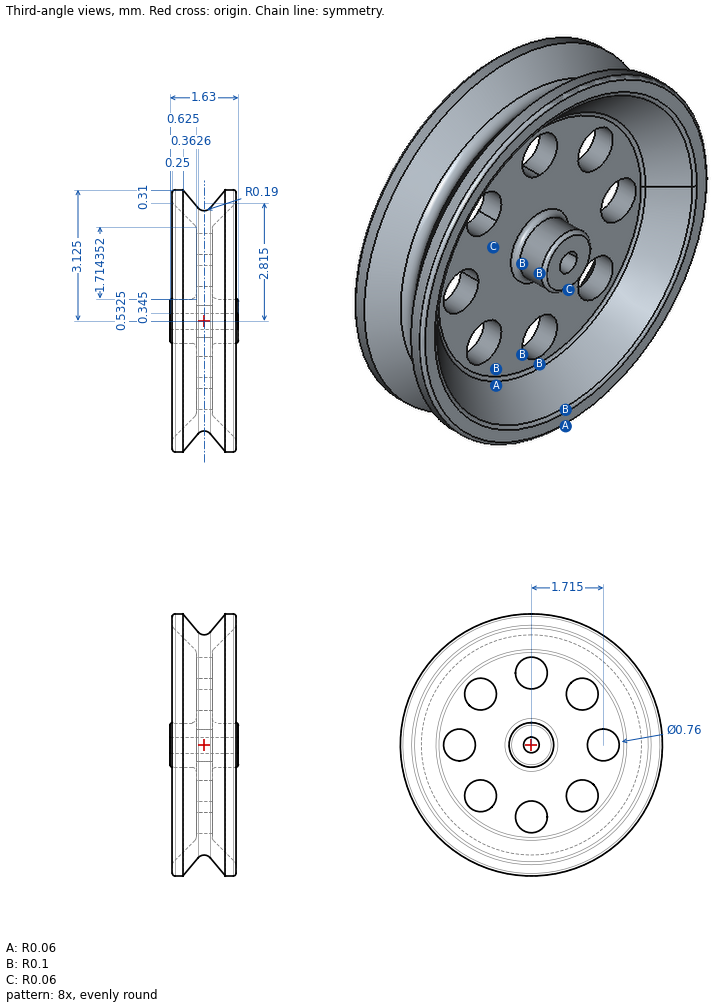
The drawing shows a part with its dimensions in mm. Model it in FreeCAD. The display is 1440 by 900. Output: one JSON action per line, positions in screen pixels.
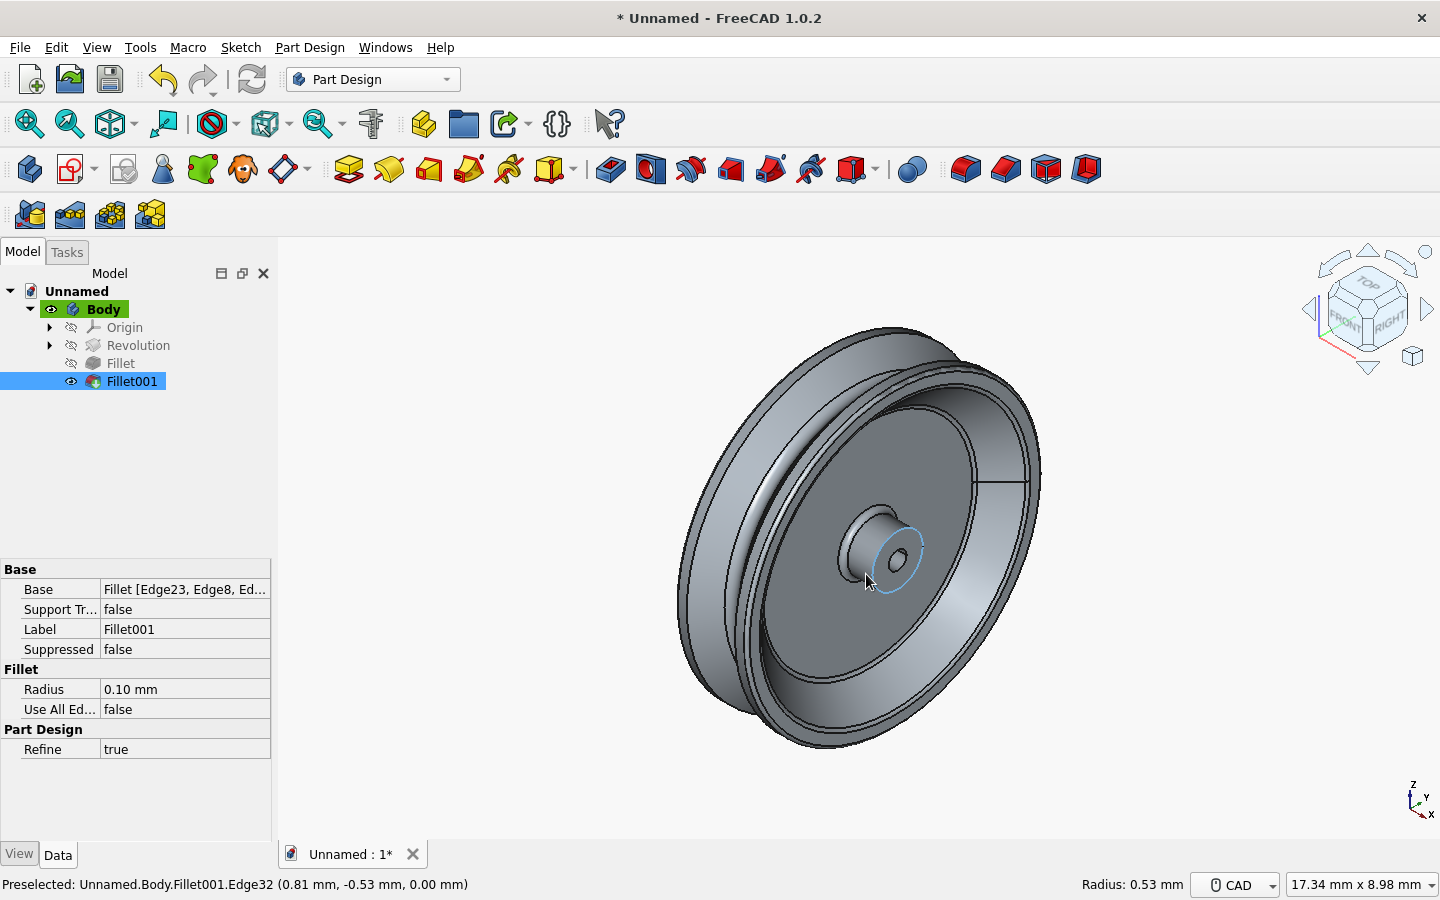
{"action": "key", "text": "2"}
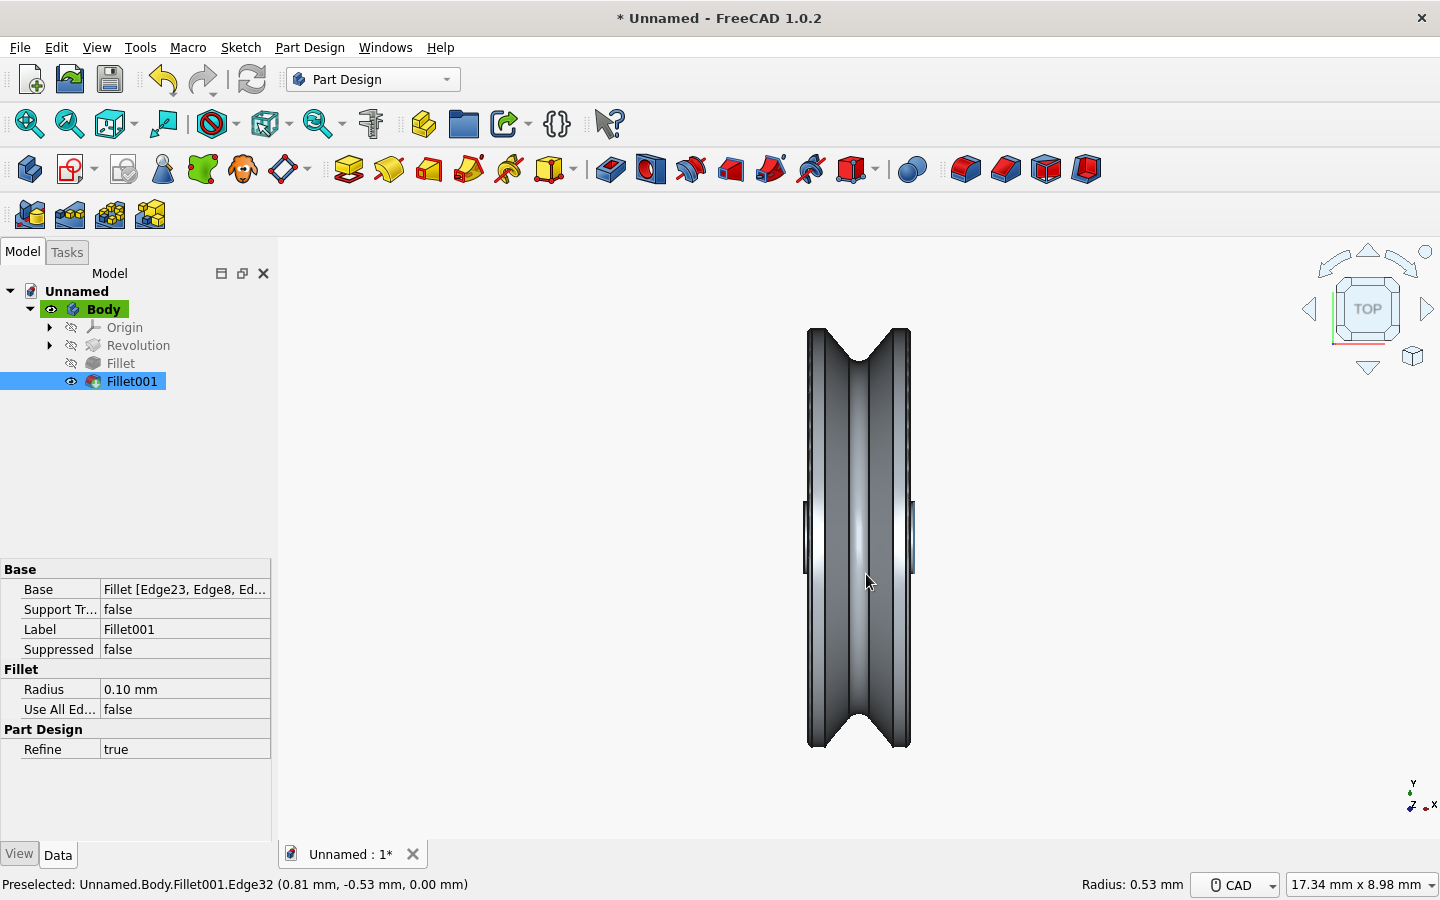
{"action": "key", "text": "0"}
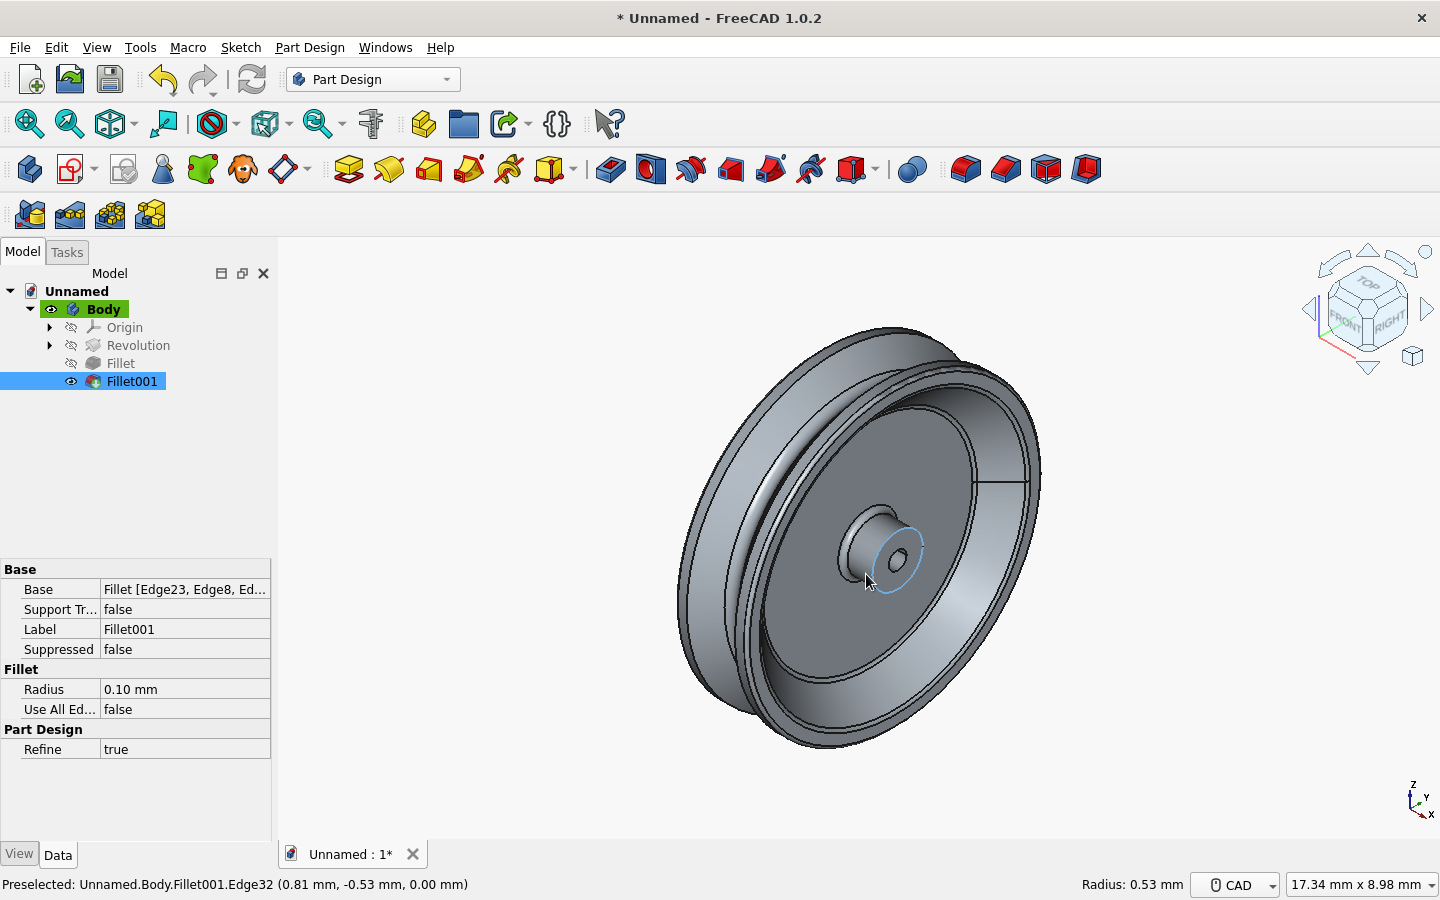
{"action": "key", "text": "1"}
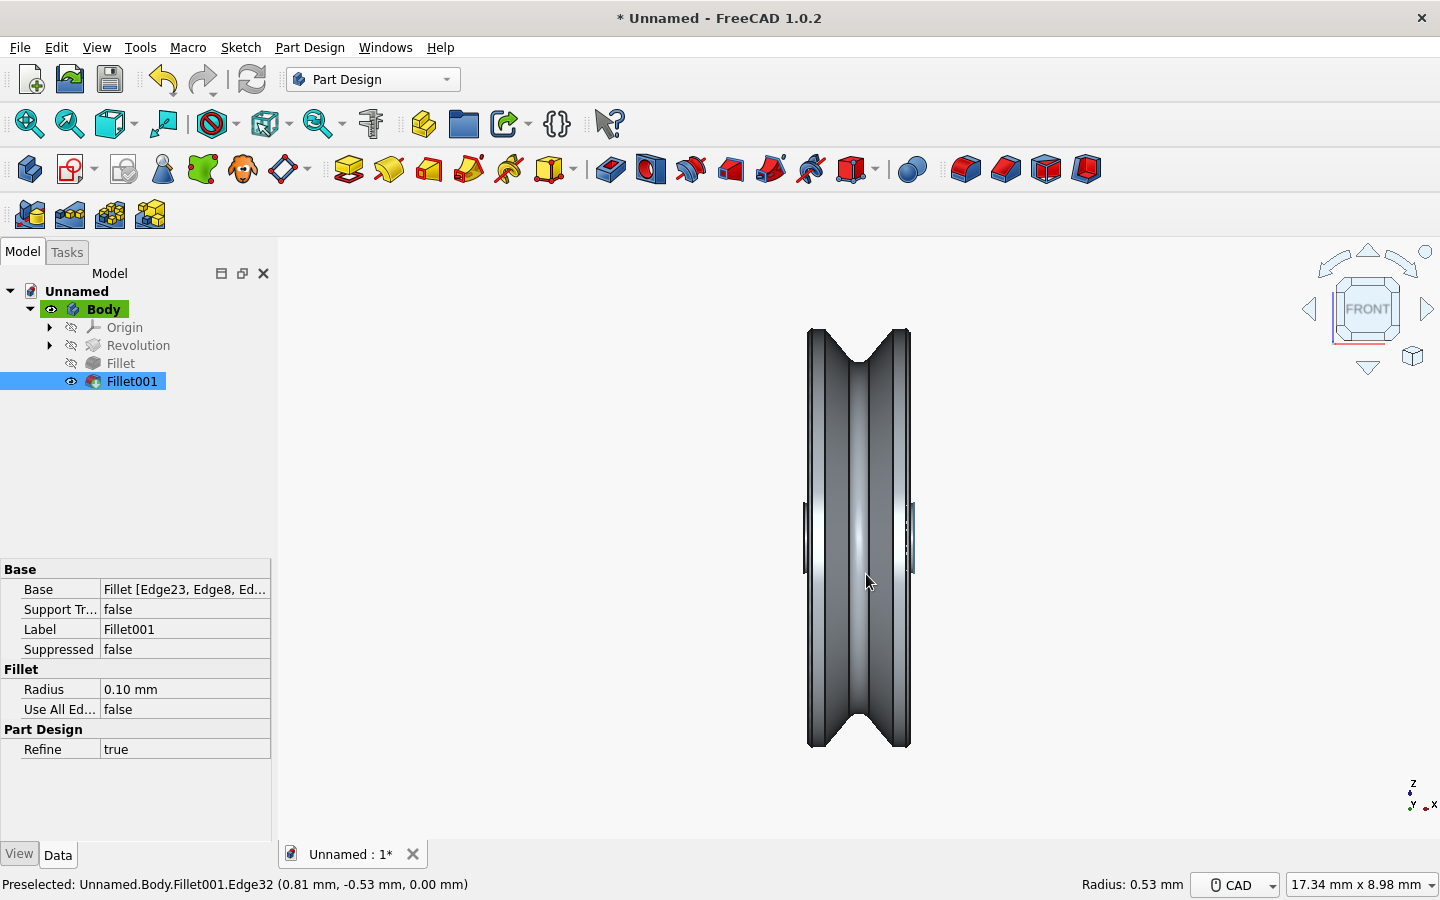
{"action": "key", "text": "3"}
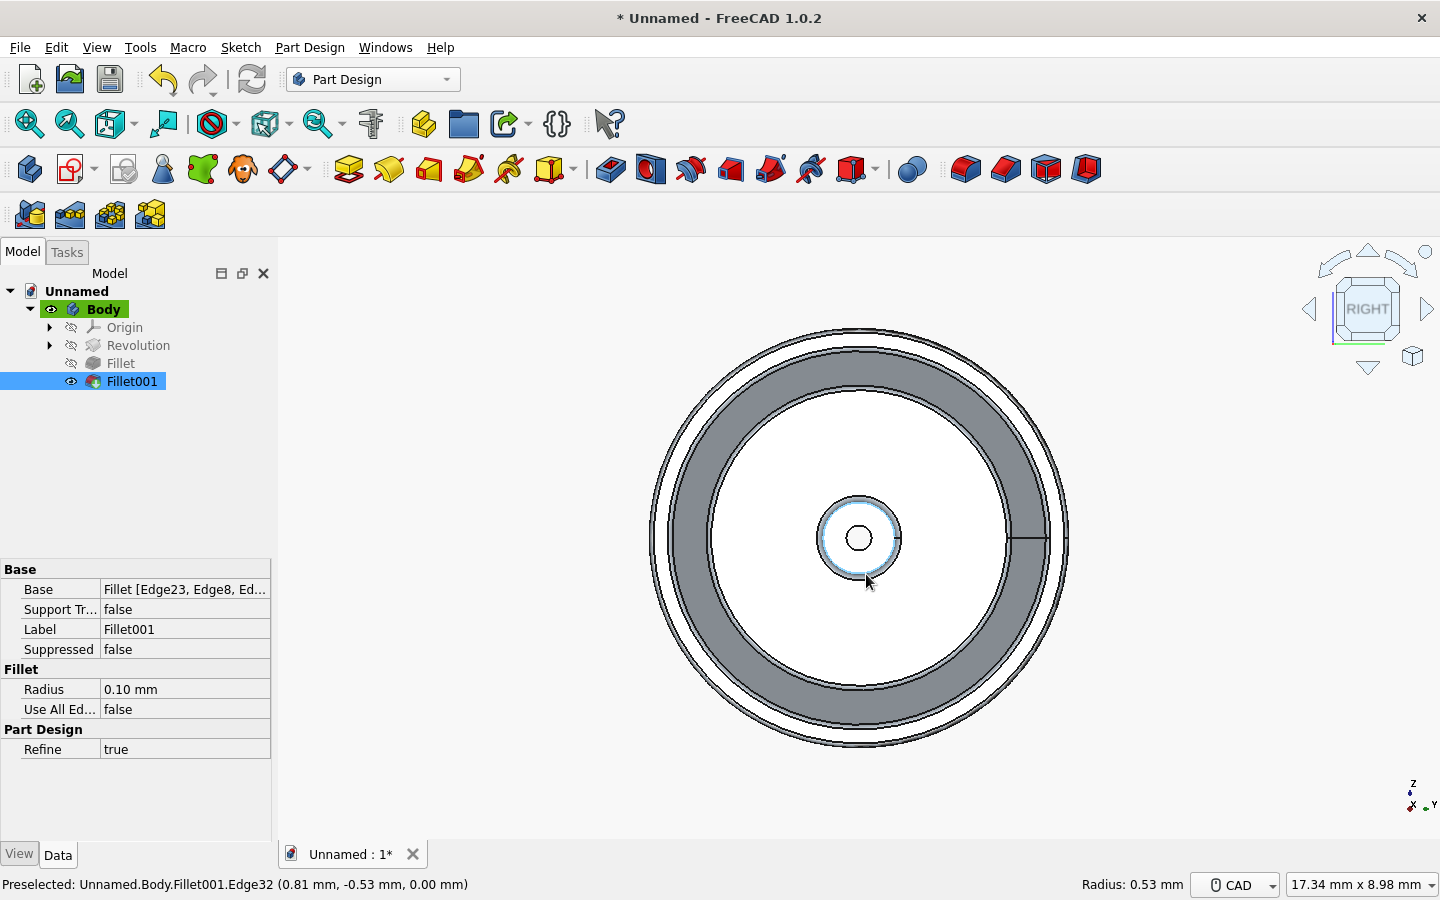
{"action": "key", "text": "5"}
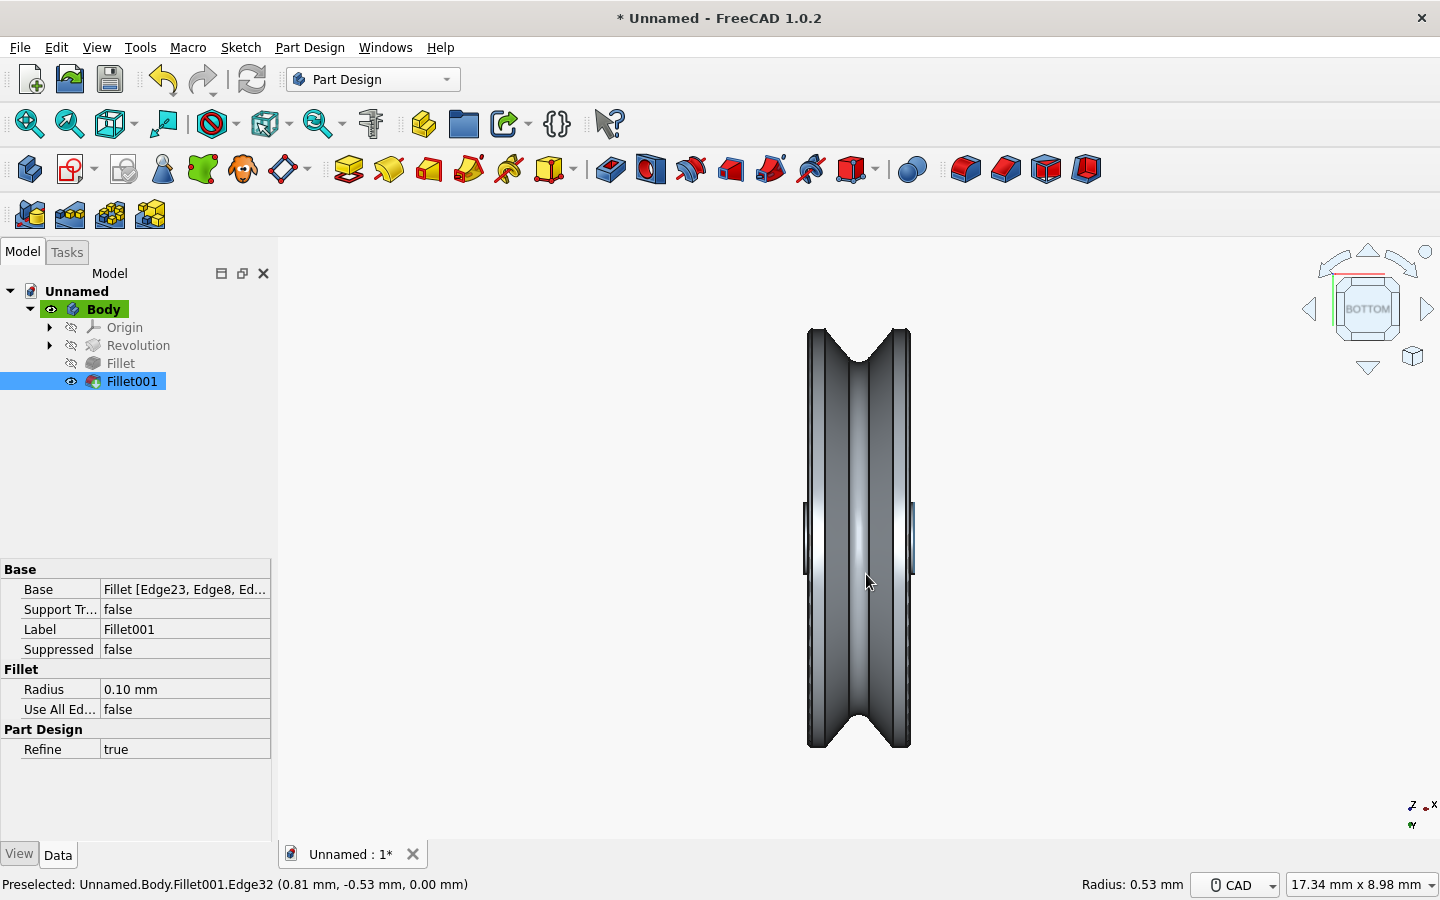
{"action": "key", "text": "4"}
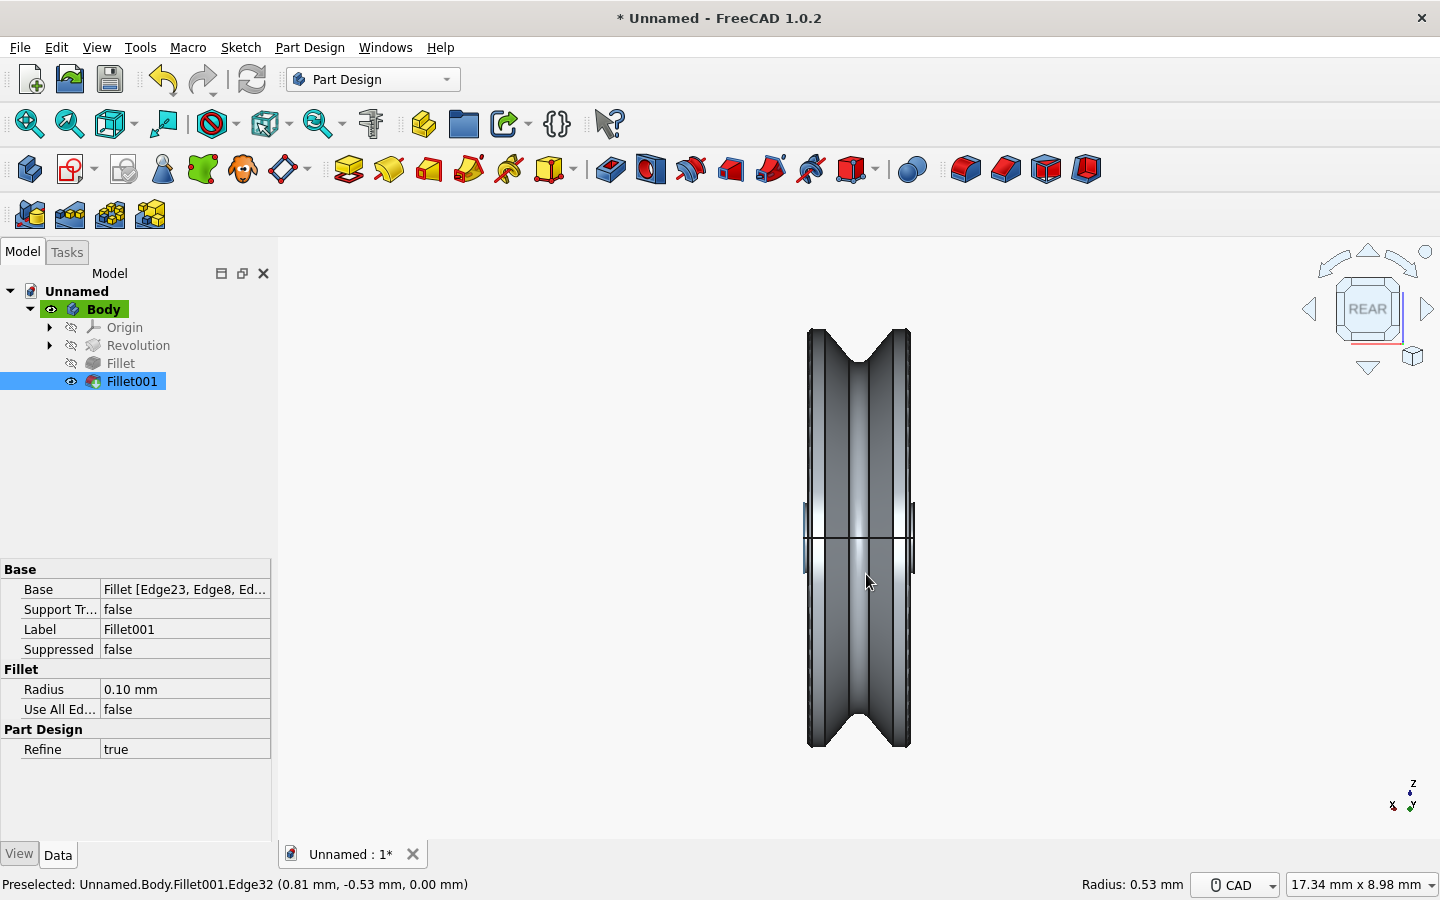
{"action": "key", "text": "6"}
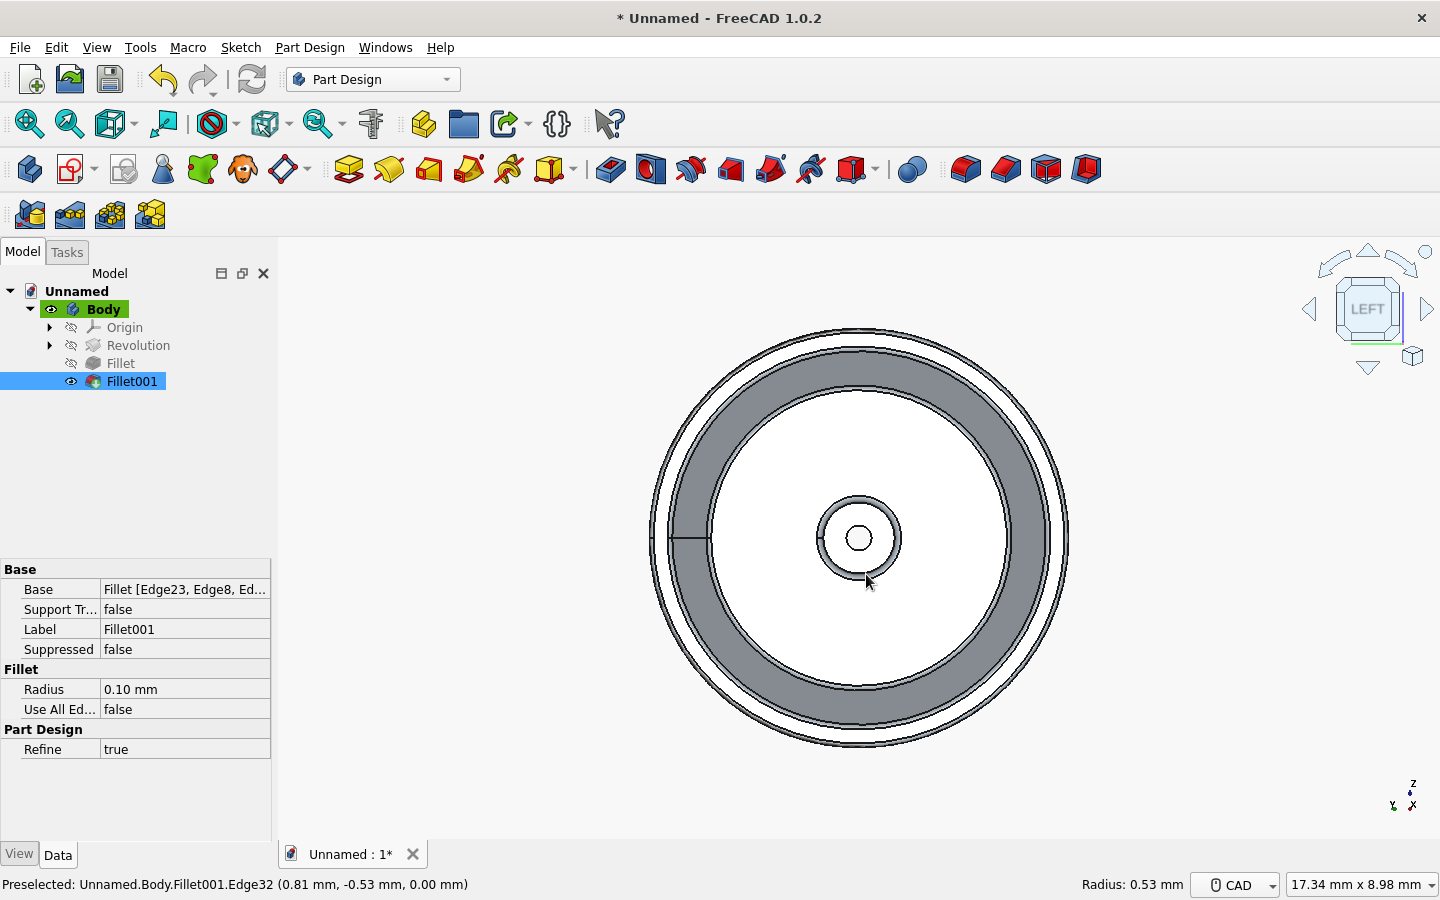
{"action": "left_click", "coordinate": [895, 537], "text": "ctrl"}